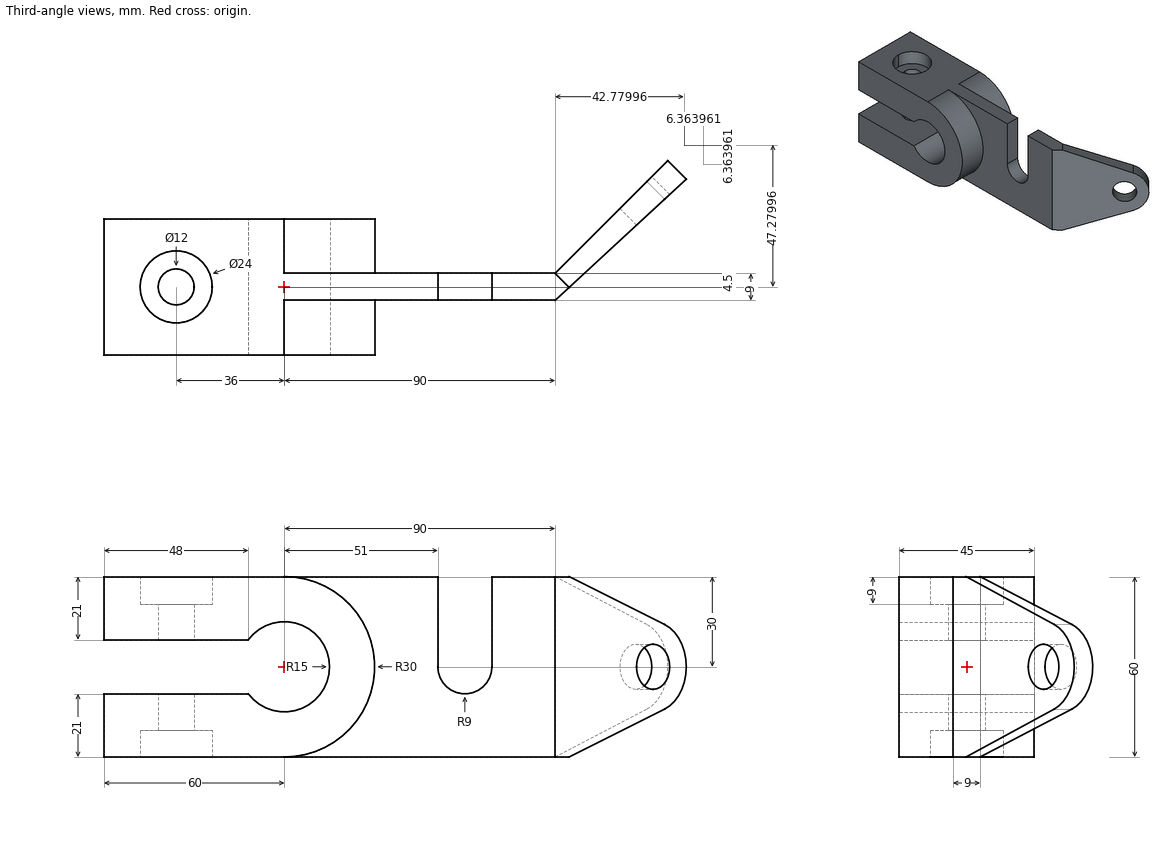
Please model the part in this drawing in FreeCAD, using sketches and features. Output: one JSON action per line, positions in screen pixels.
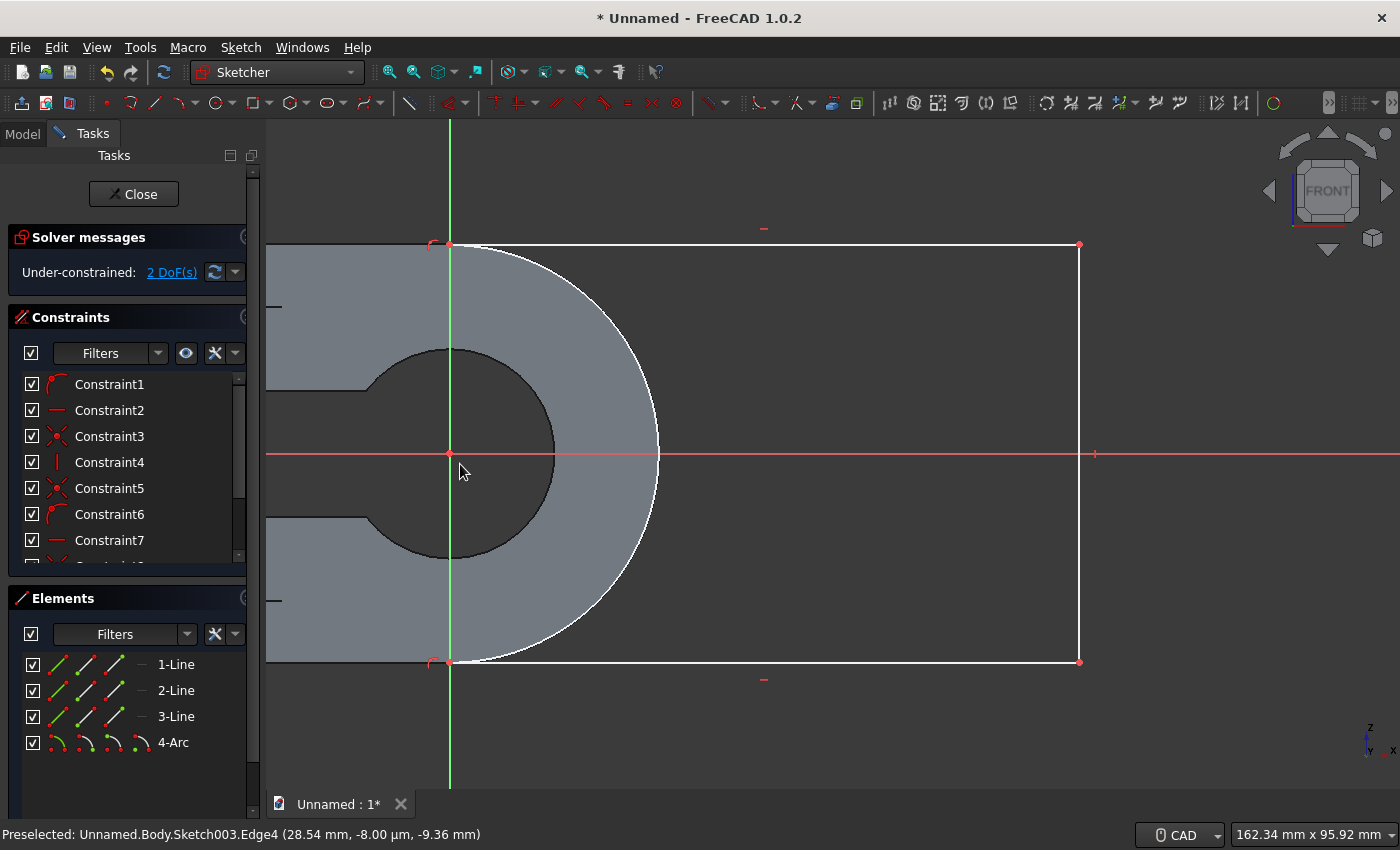
{"action": "key", "text": "d"}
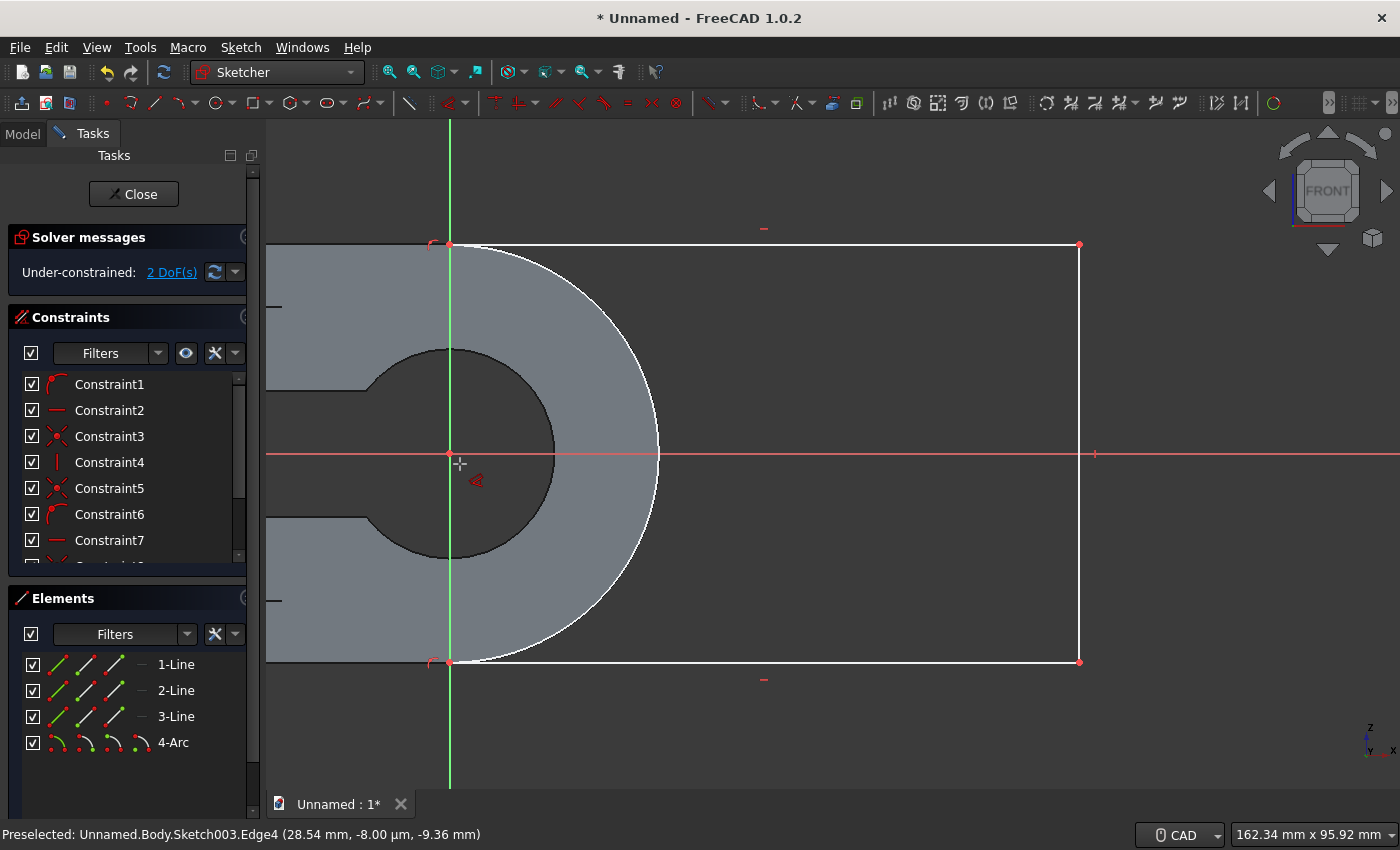
{"action": "left_click", "coordinate": [619, 577]}
{"action": "left_click", "coordinate": [645, 596]}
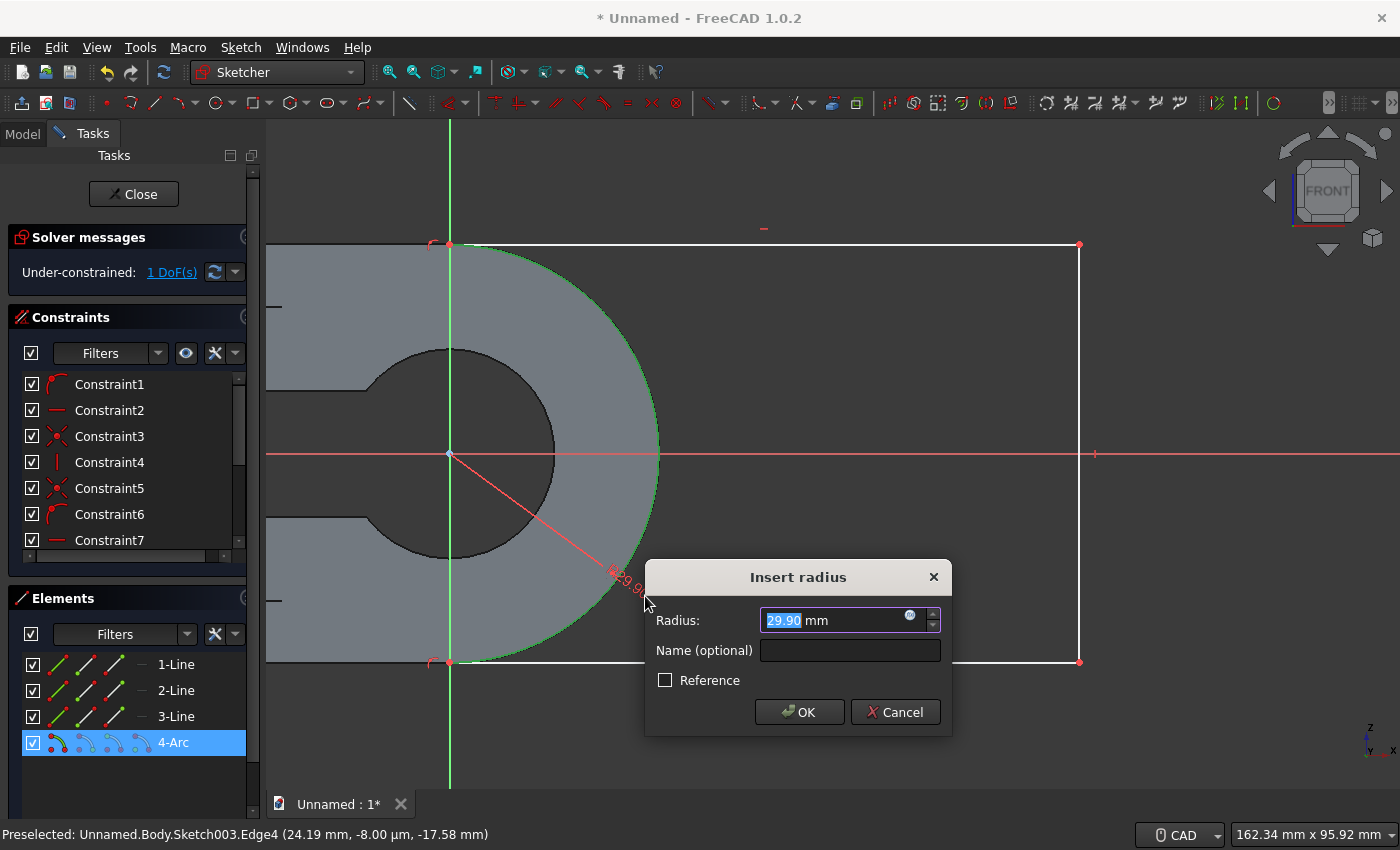
{"action": "type", "text": "30"}
{"action": "key", "text": "Return"}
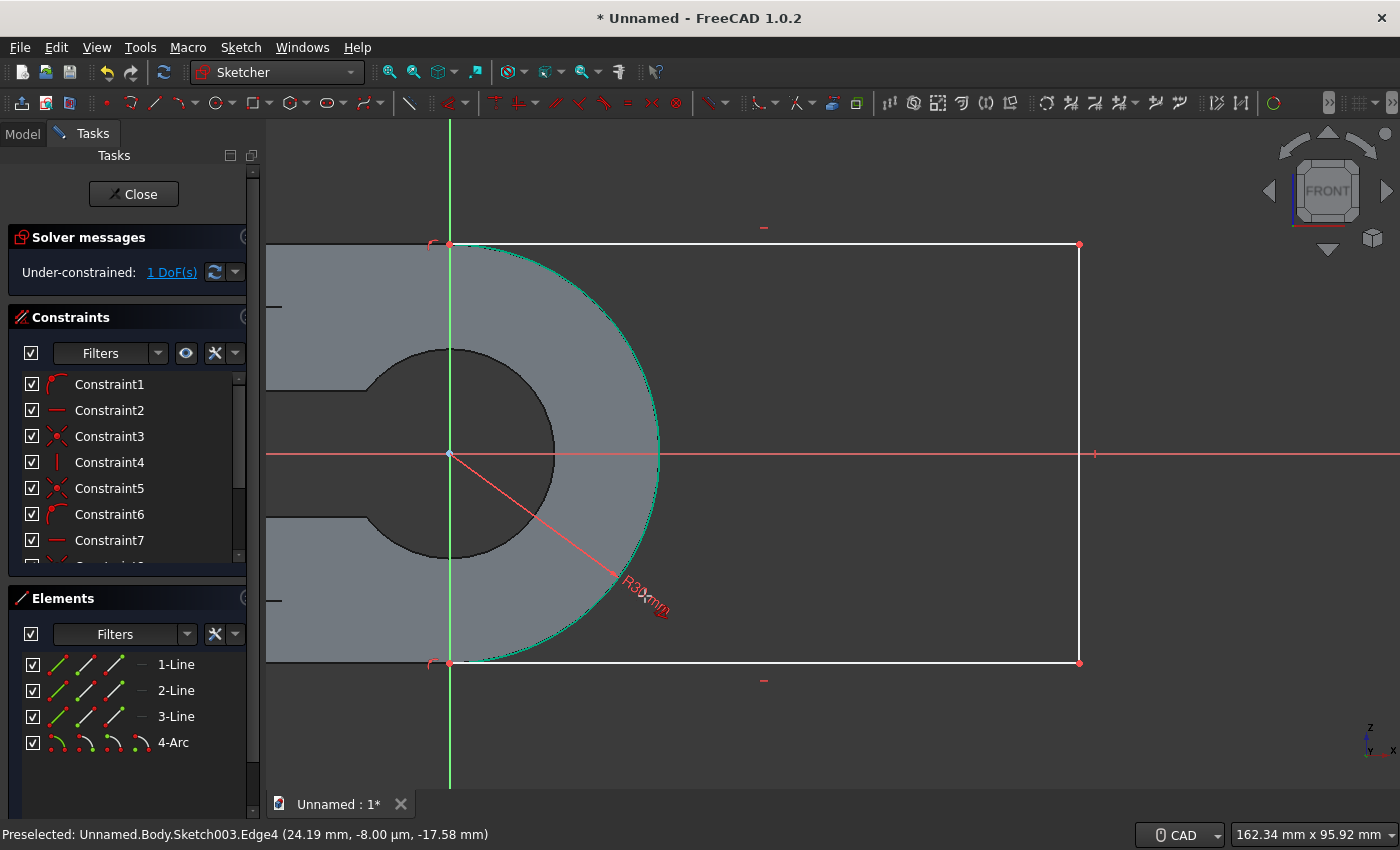
{"action": "left_click", "coordinate": [639, 244]}
{"action": "left_click", "coordinate": [764, 210]}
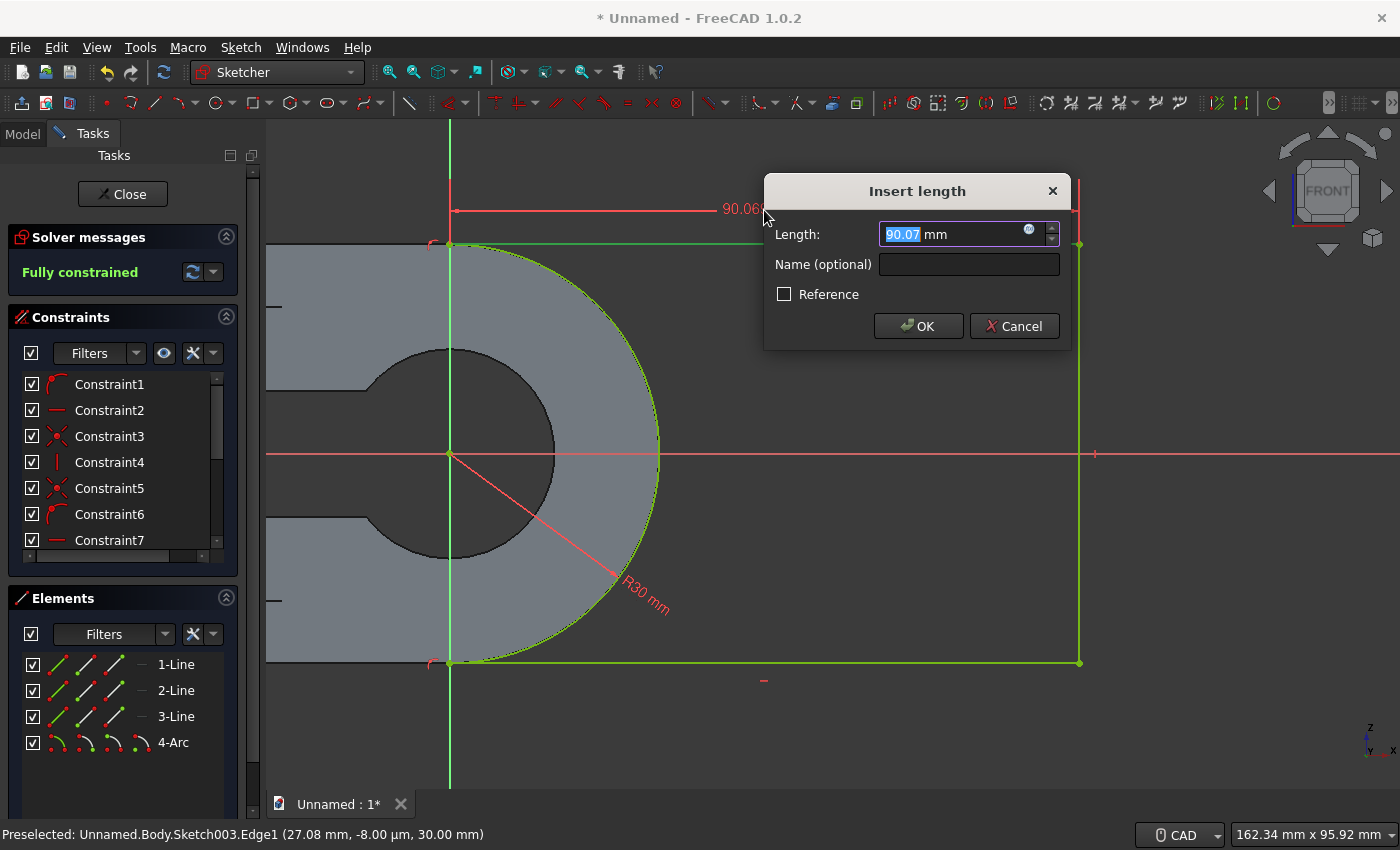
{"action": "type", "text": "90"}
{"action": "key", "text": "Return"}
{"action": "key", "text": "Escape"}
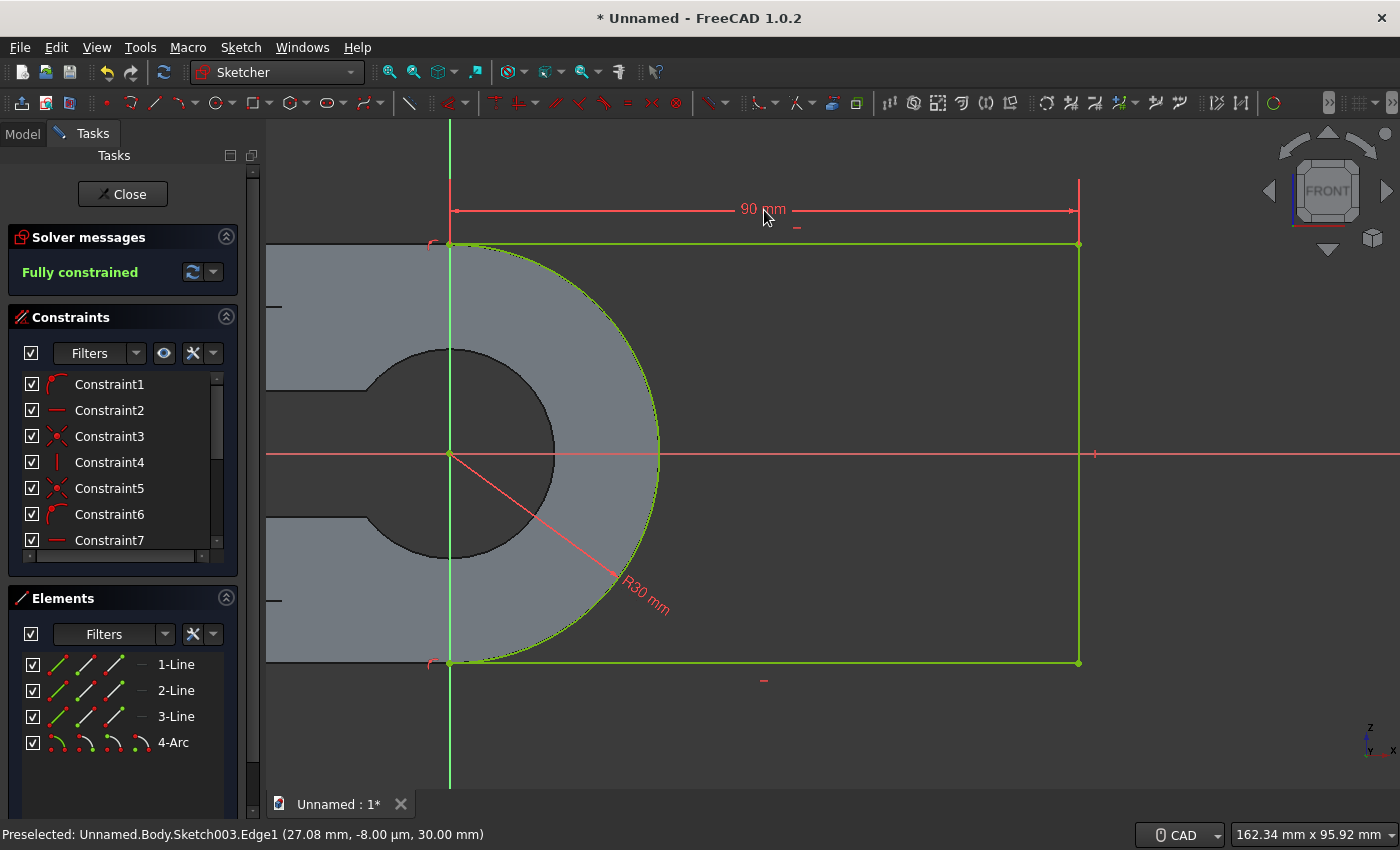
{"action": "left_click", "coordinate": [123, 194]}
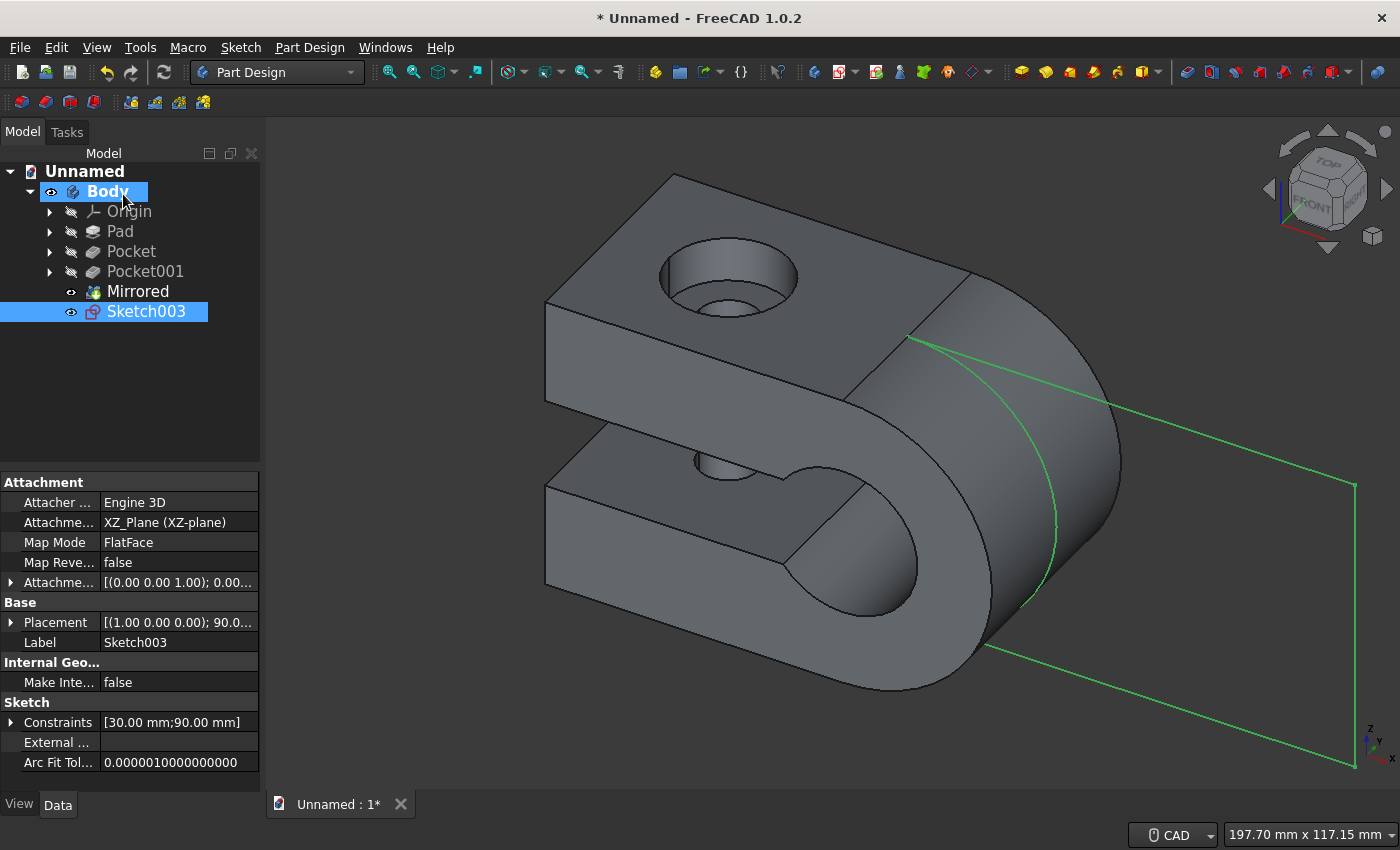
{"action": "left_click", "coordinate": [1022, 72]}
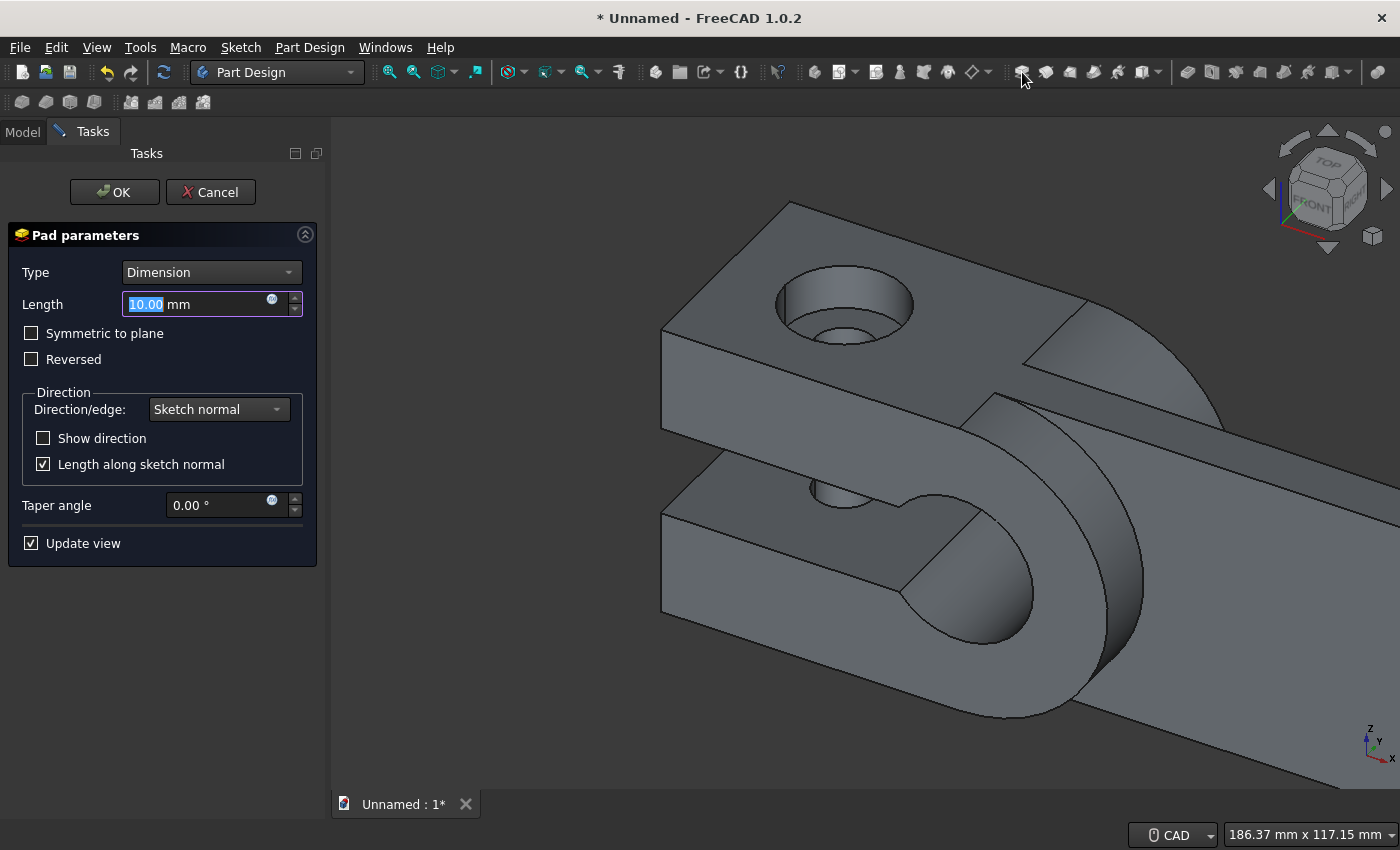
{"action": "type", "text": "9"}
{"action": "key", "text": "Tab"}